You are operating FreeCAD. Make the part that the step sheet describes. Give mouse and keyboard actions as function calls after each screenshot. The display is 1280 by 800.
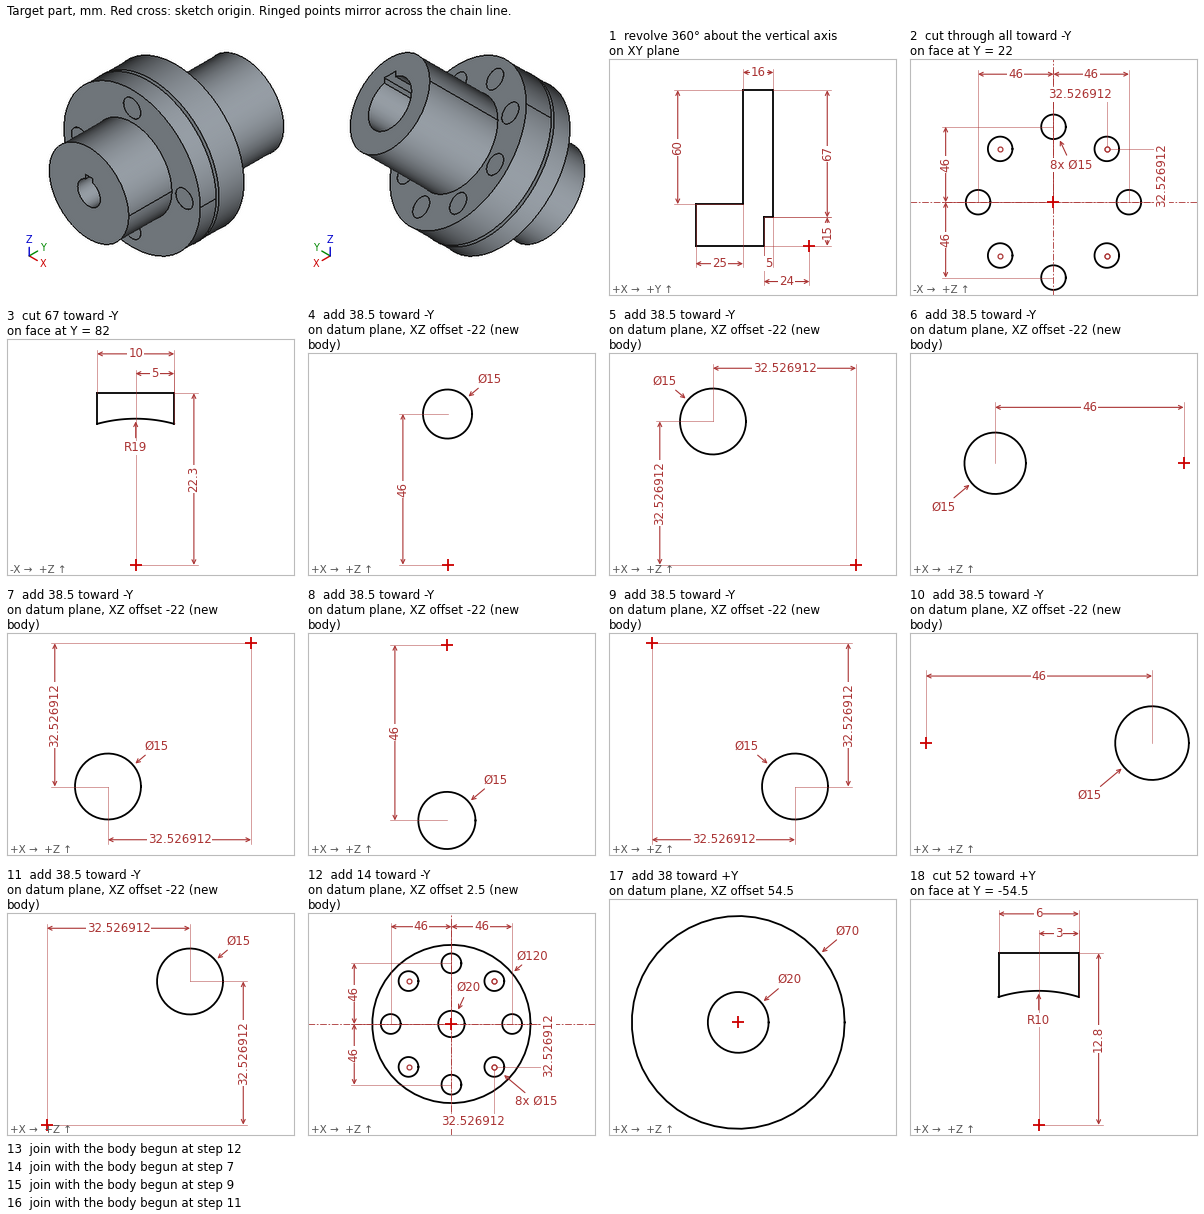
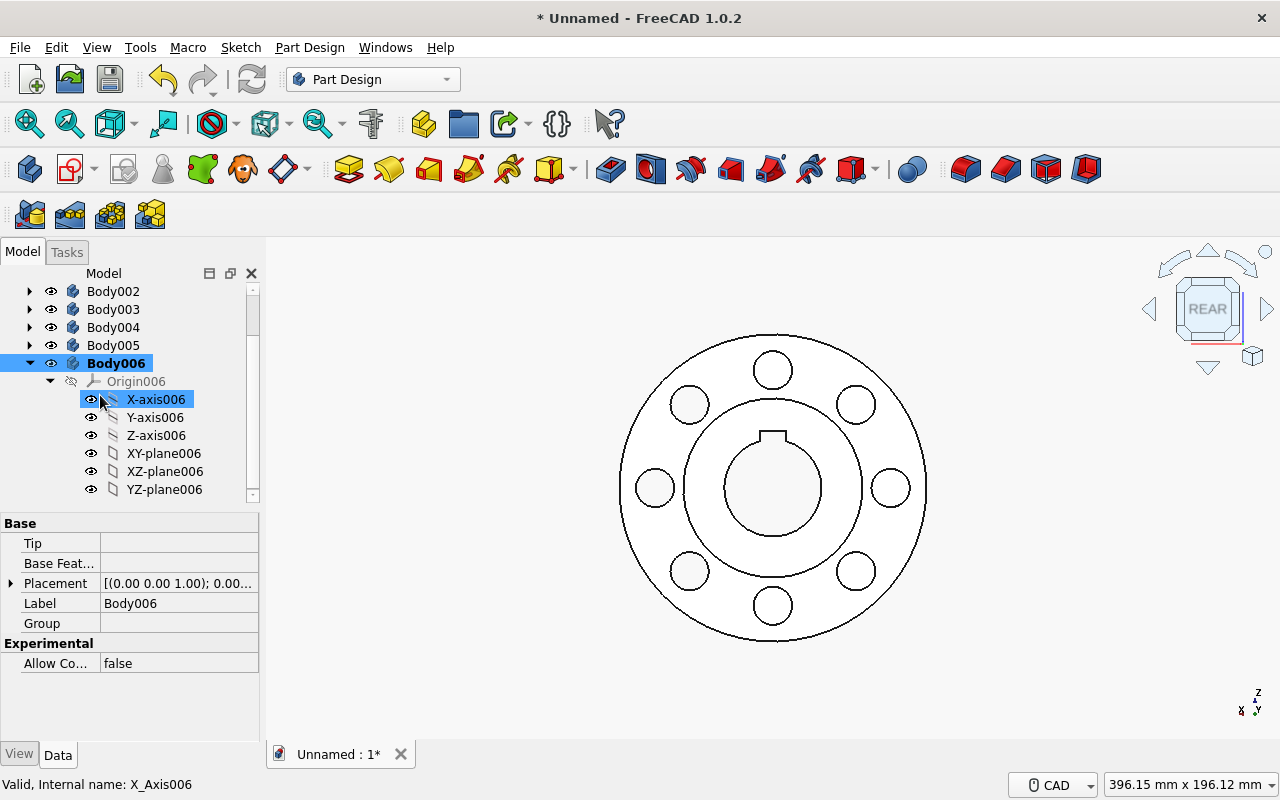
click(136, 471)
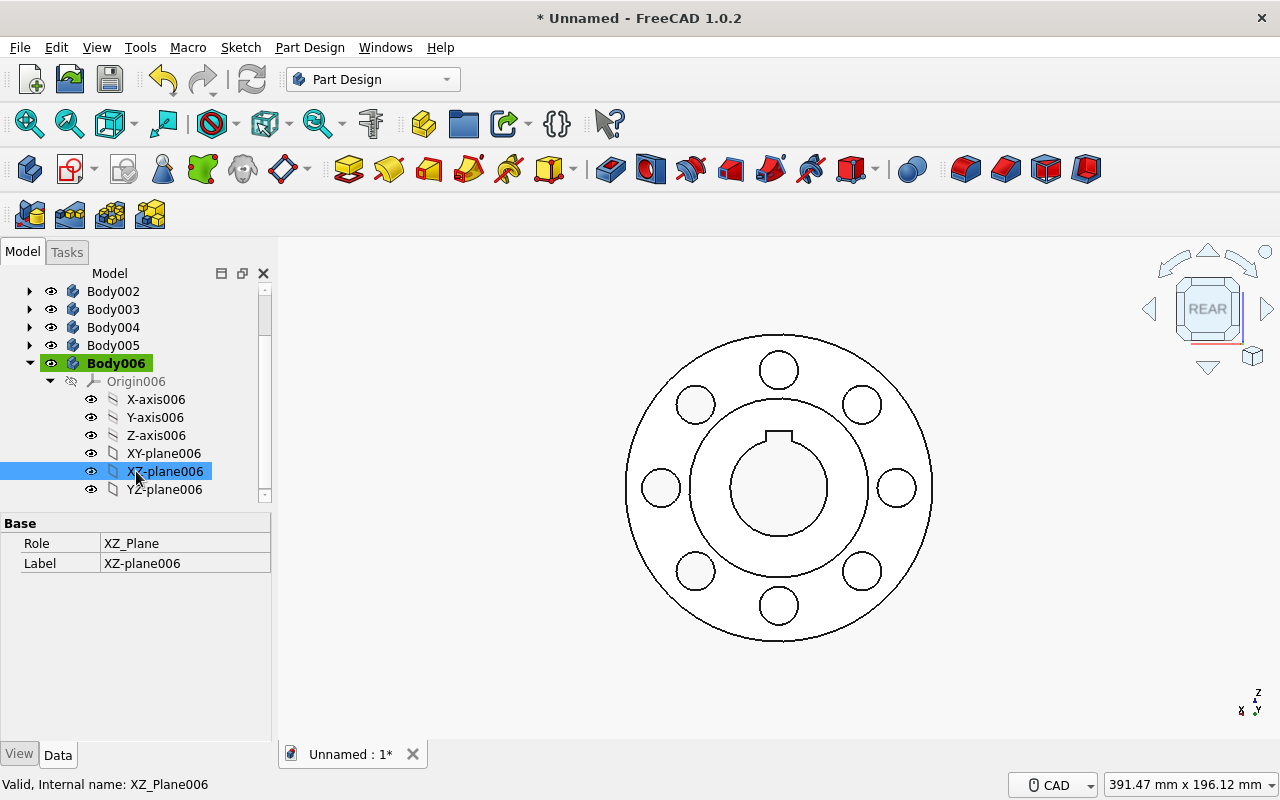
click(284, 170)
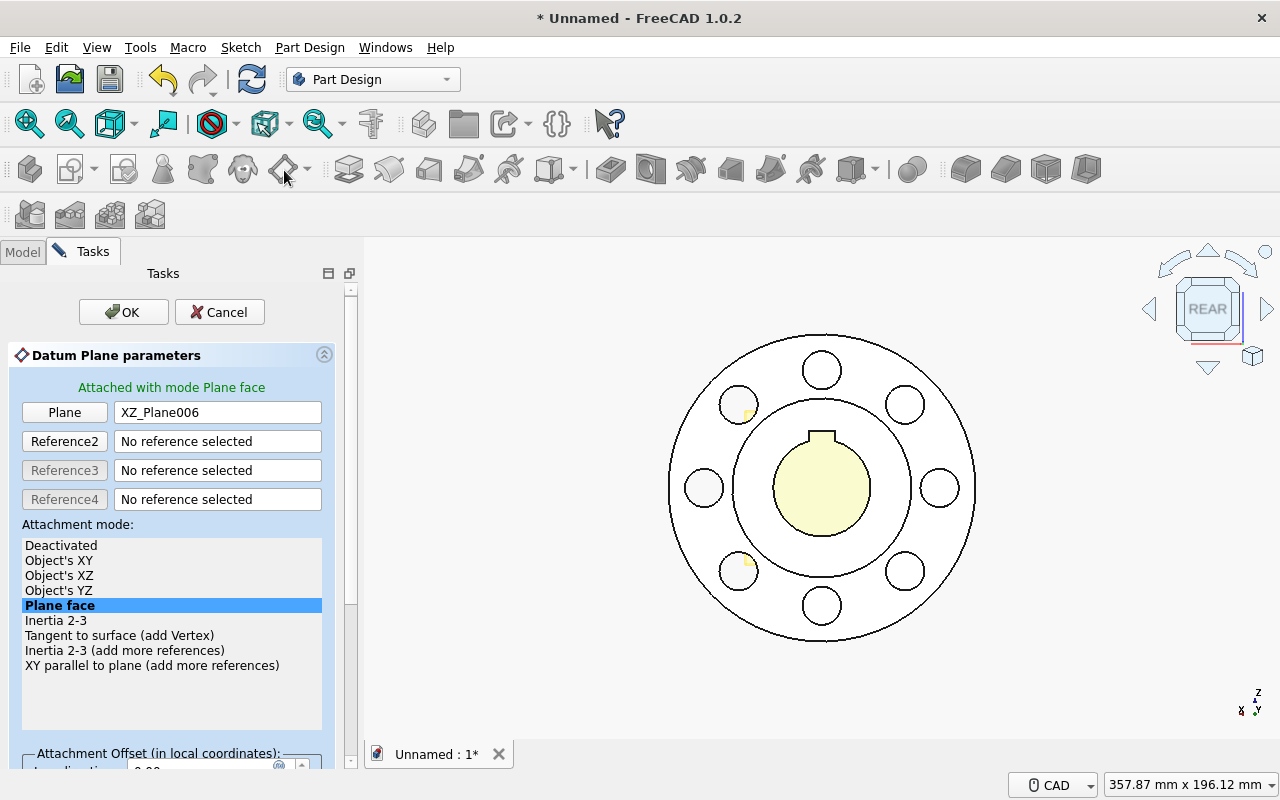
scroll(351, 526, down, 3)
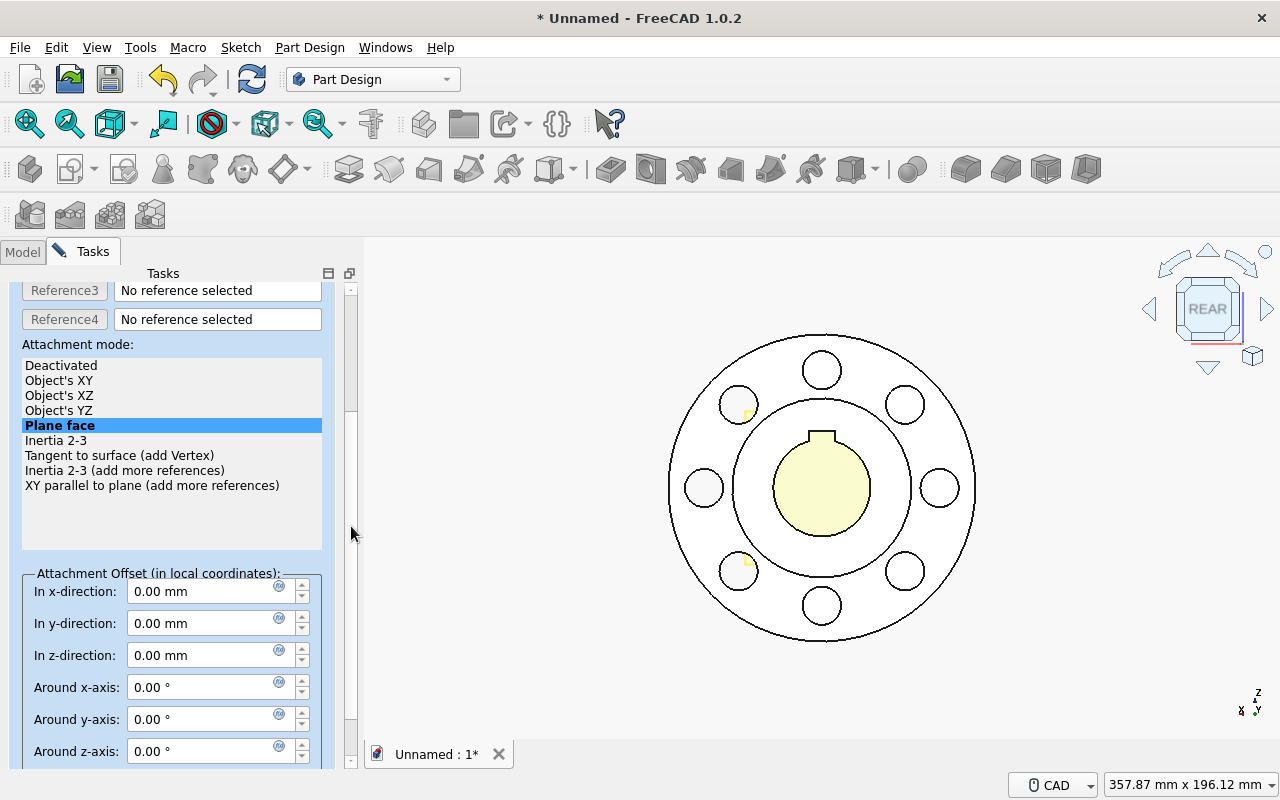
triple_click(210, 655)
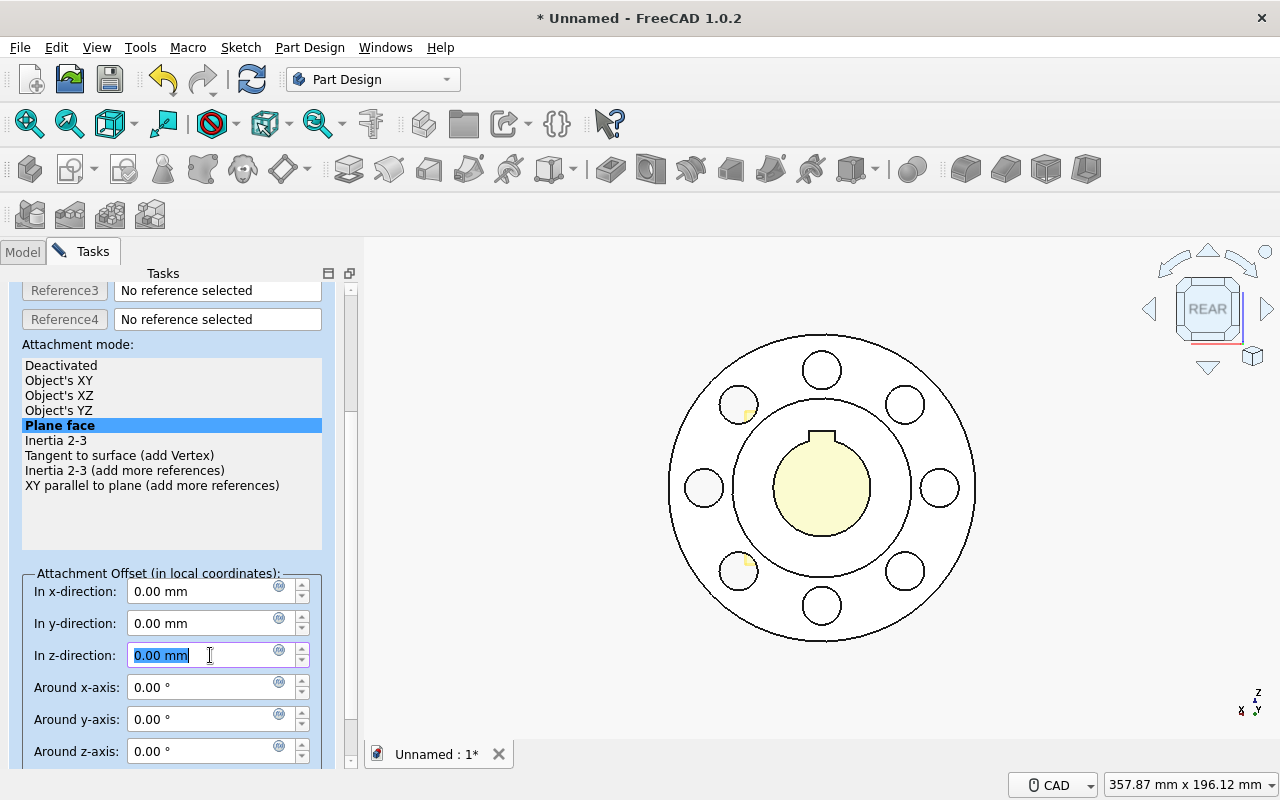
text(-22)
key(Tab)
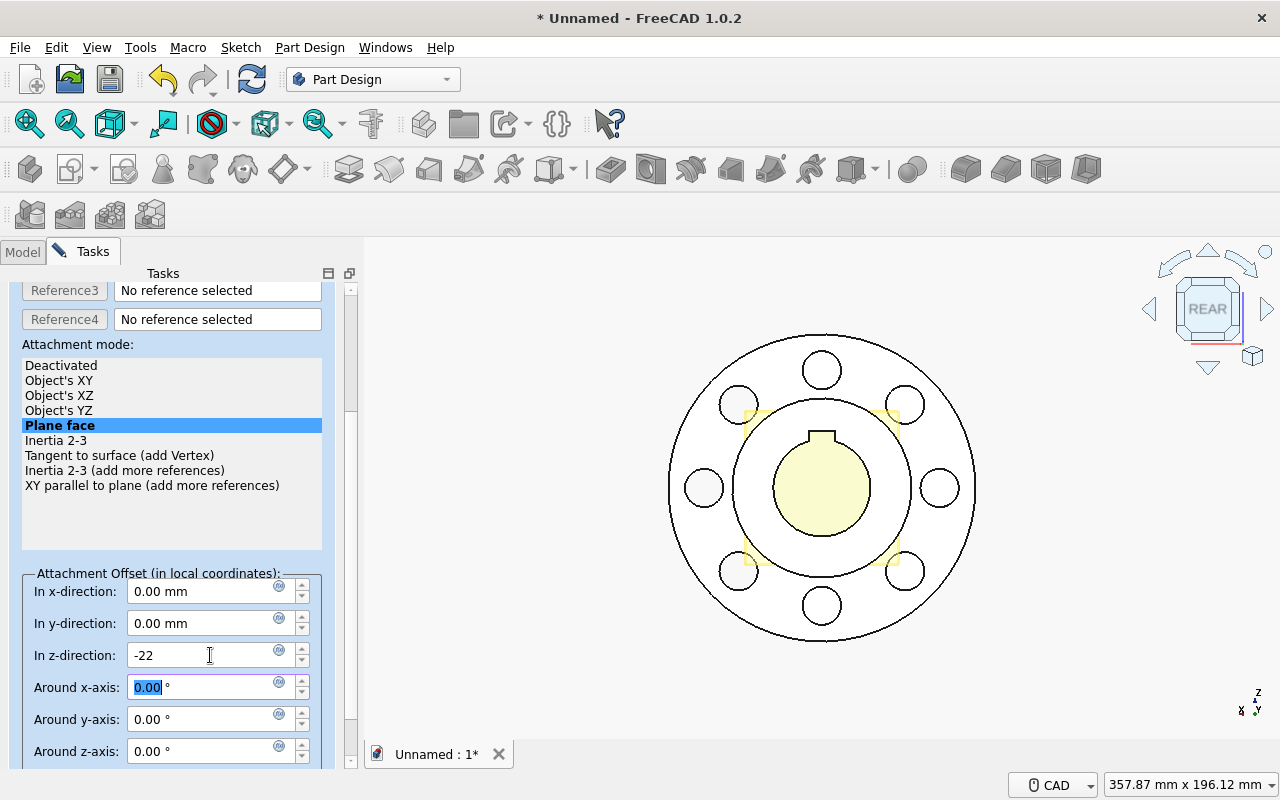
scroll(351, 526, up, 4)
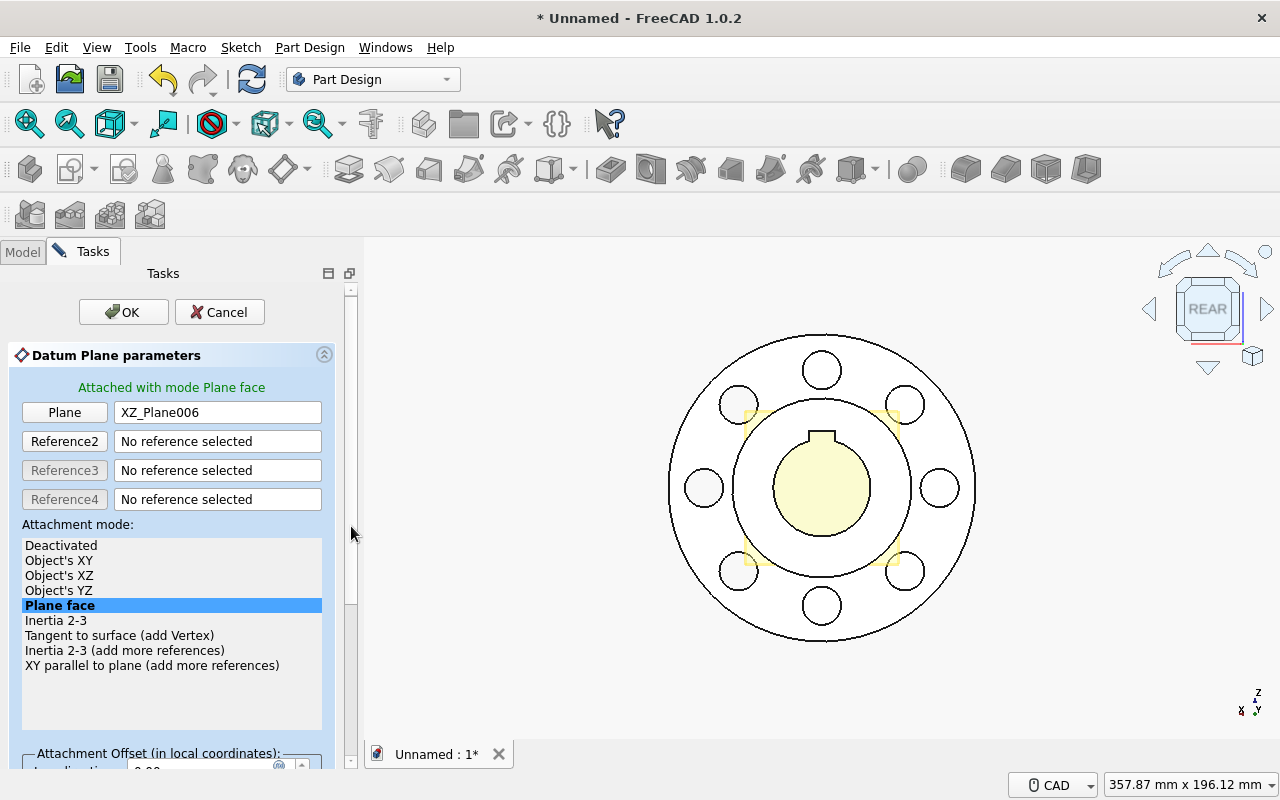
click(124, 312)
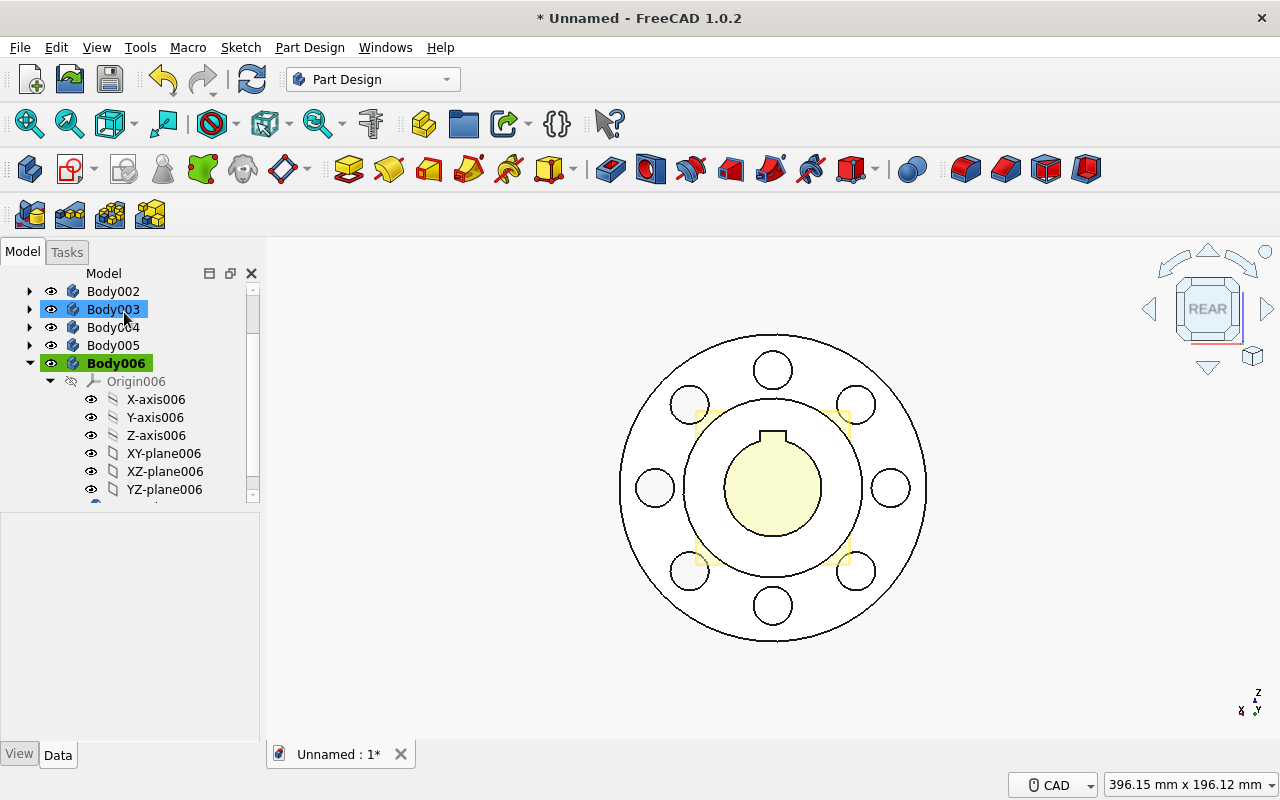
scroll(120, 395, down, 3)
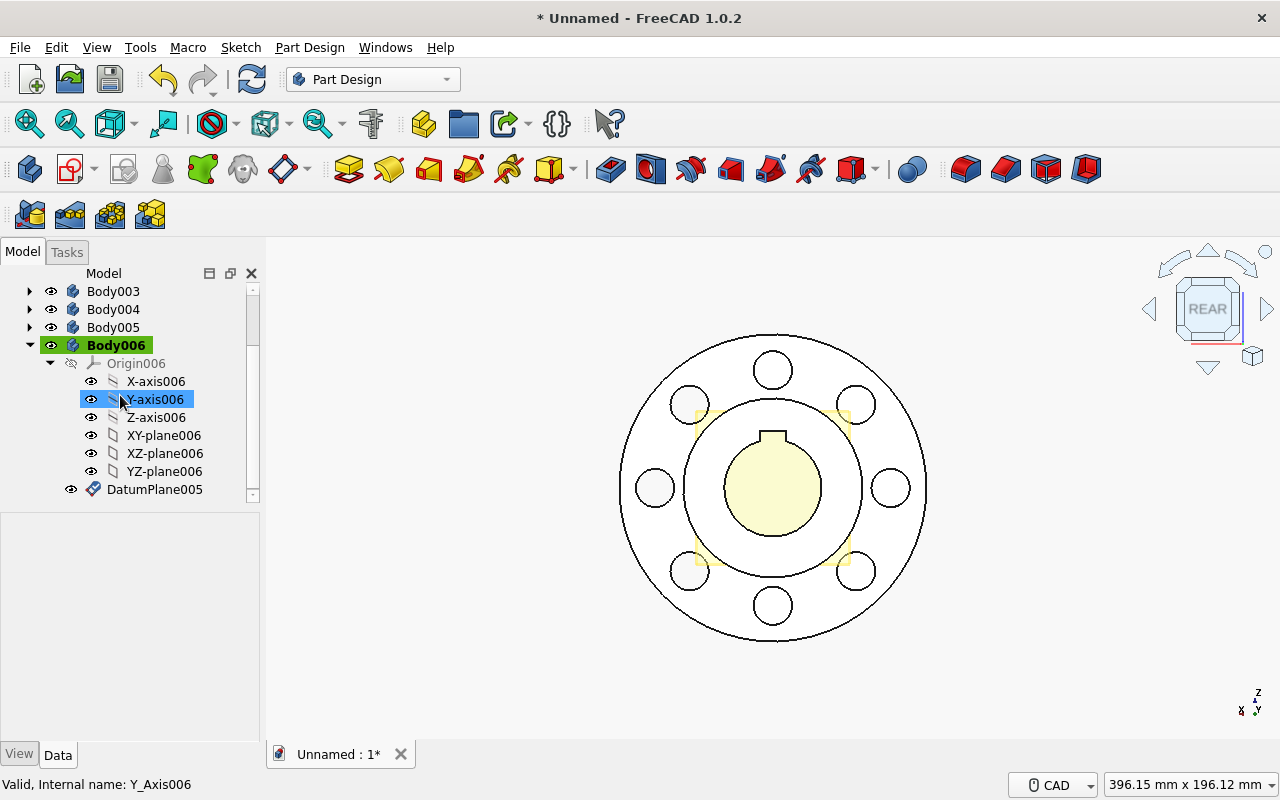
click(116, 489)